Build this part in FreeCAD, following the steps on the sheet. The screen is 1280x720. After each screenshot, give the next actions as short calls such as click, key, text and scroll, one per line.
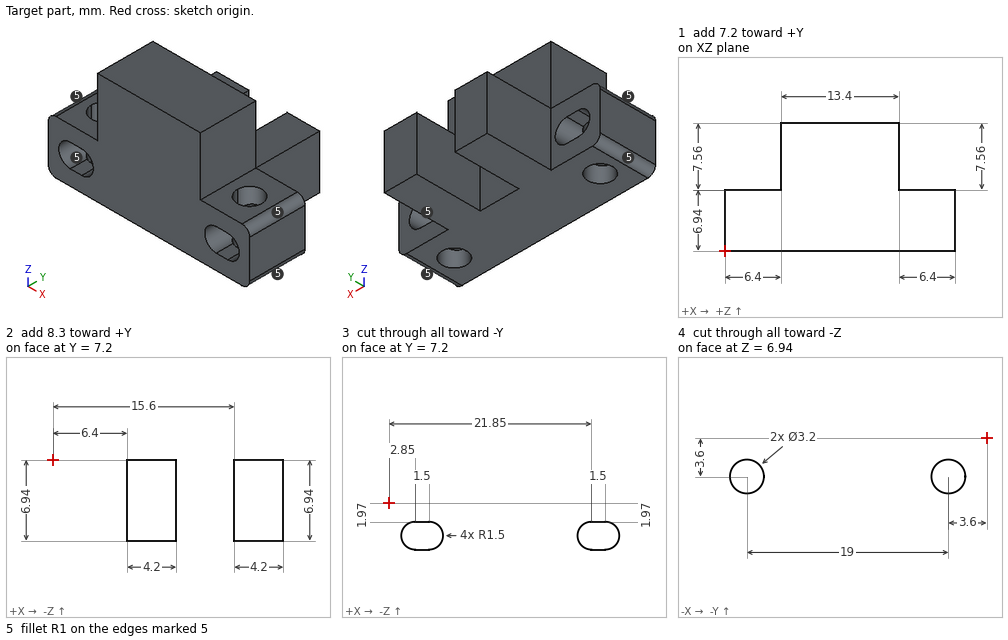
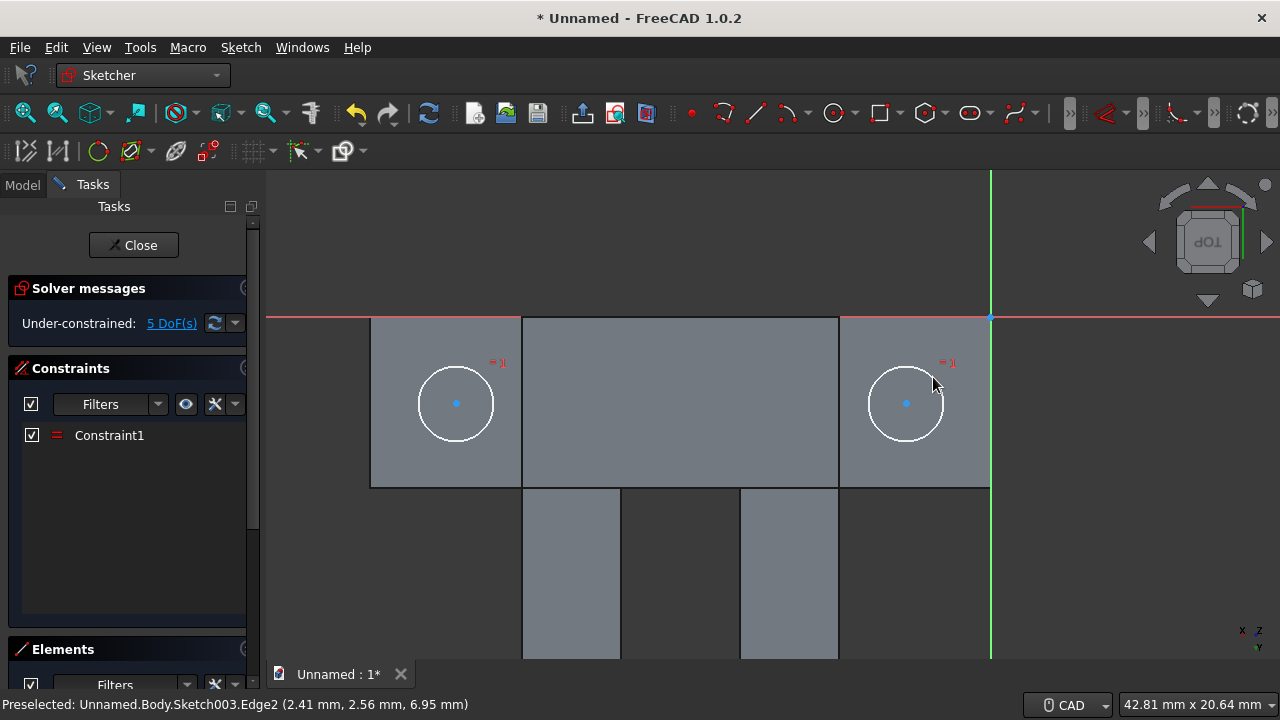
click(456, 404)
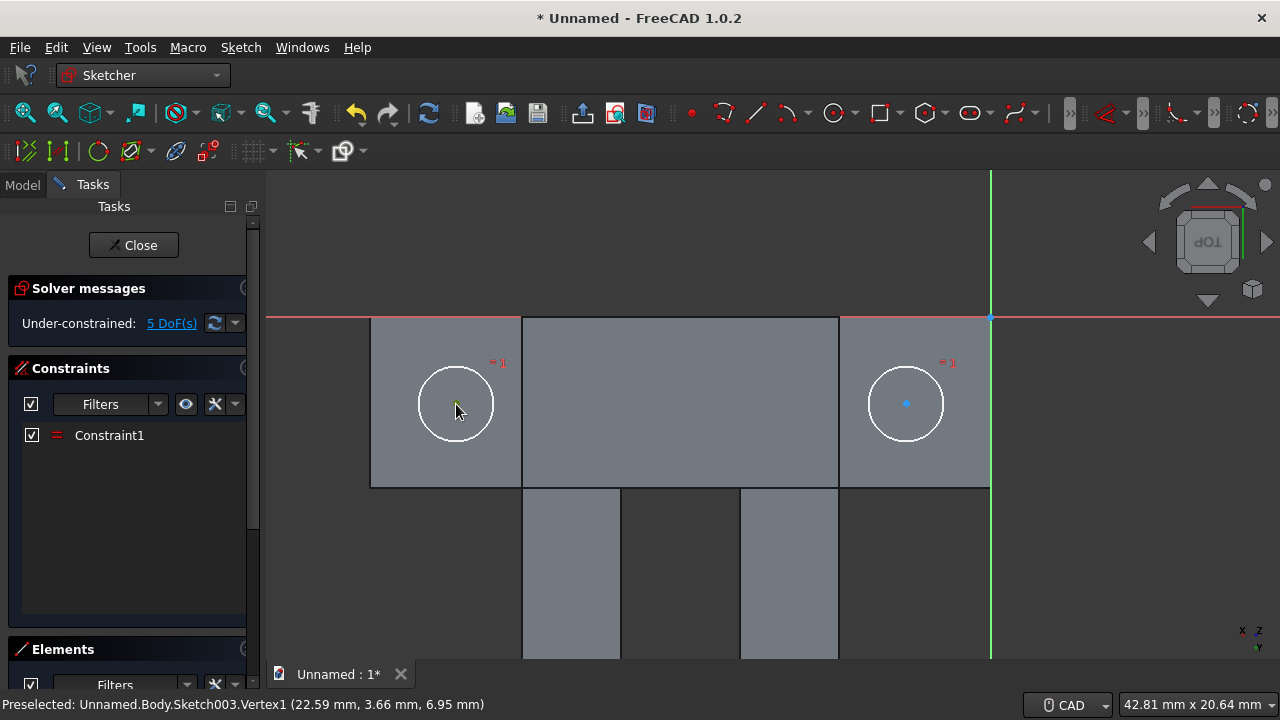
click(906, 404)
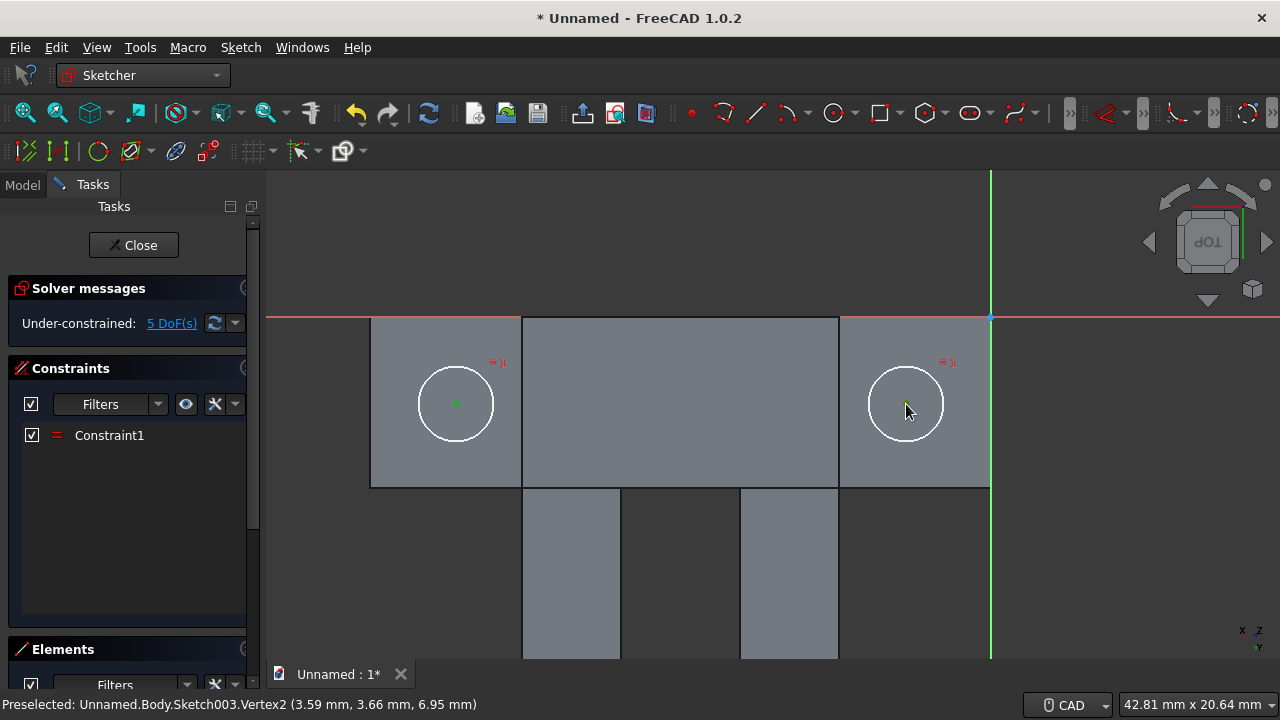
key(h)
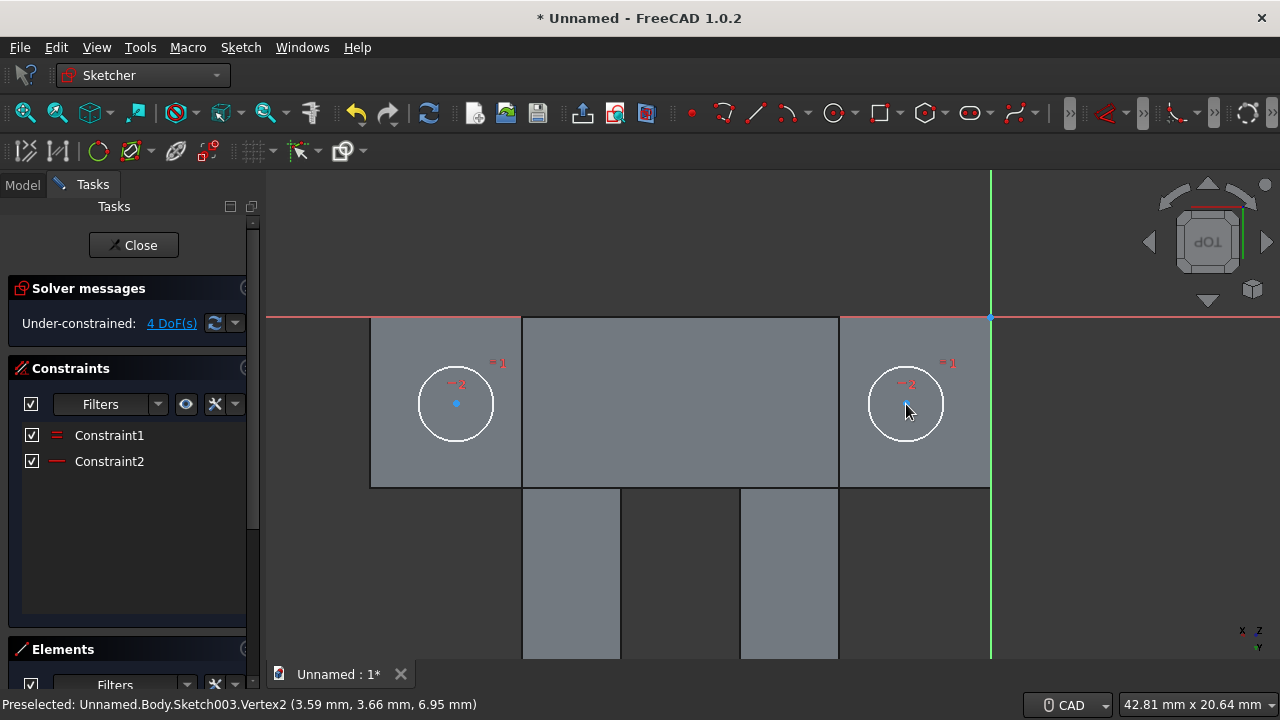
click(1106, 114)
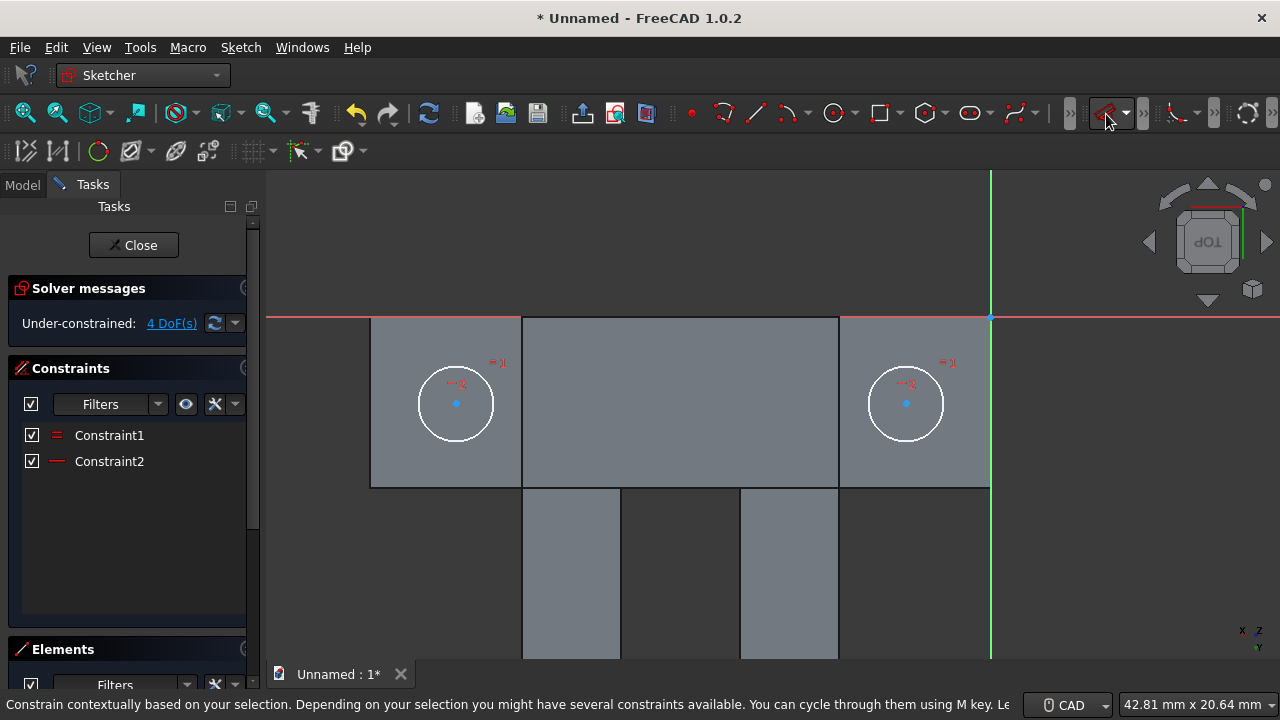
click(482, 377)
click(504, 354)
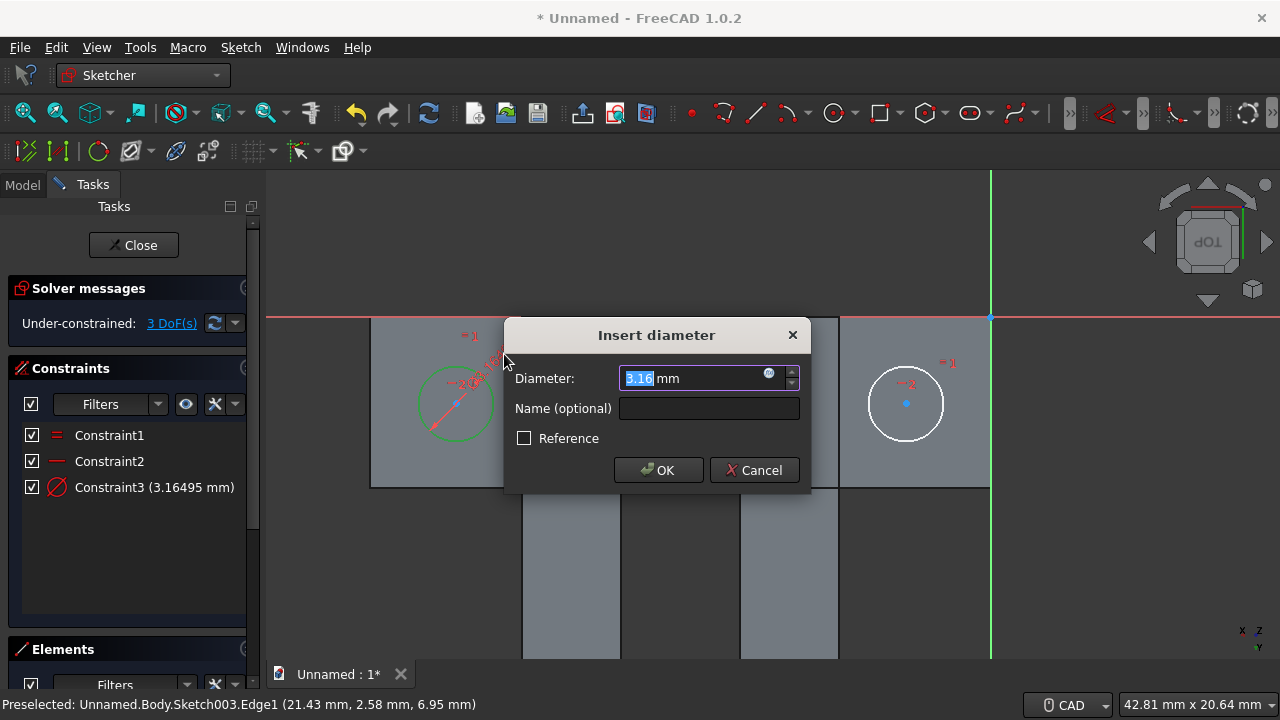
text(3.2)
key(Return)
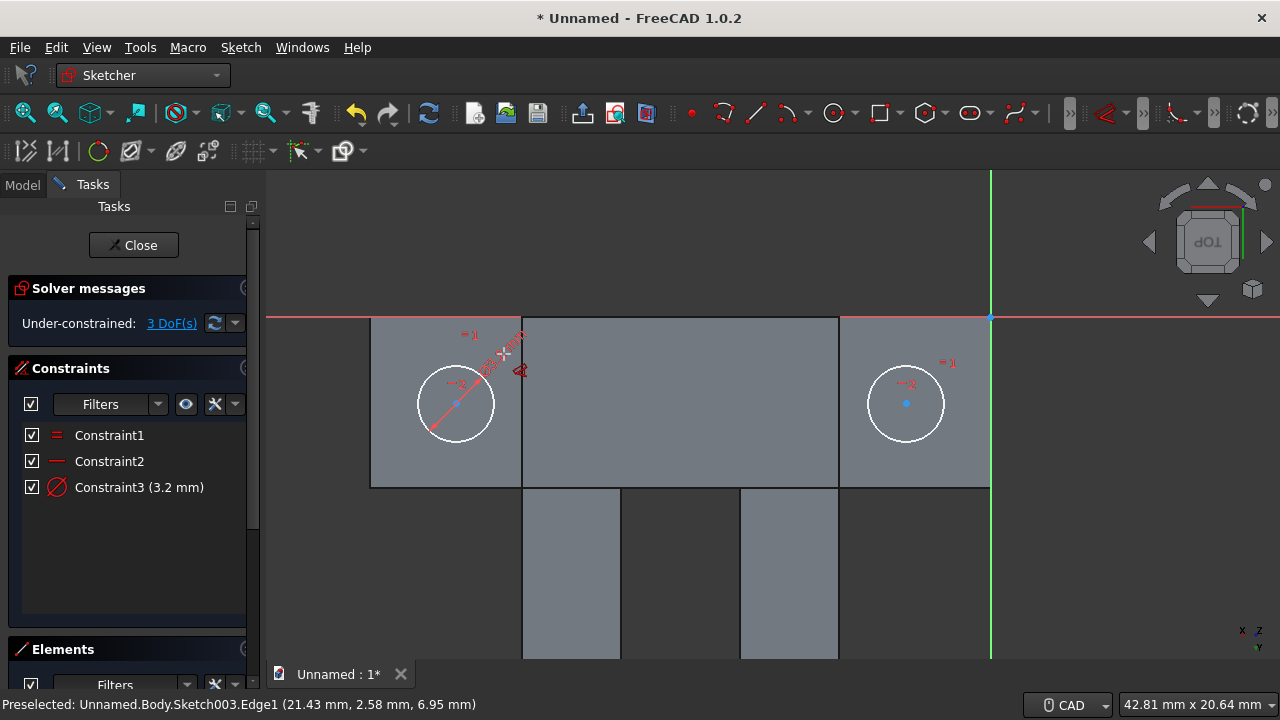
click(456, 404)
click(1025, 361)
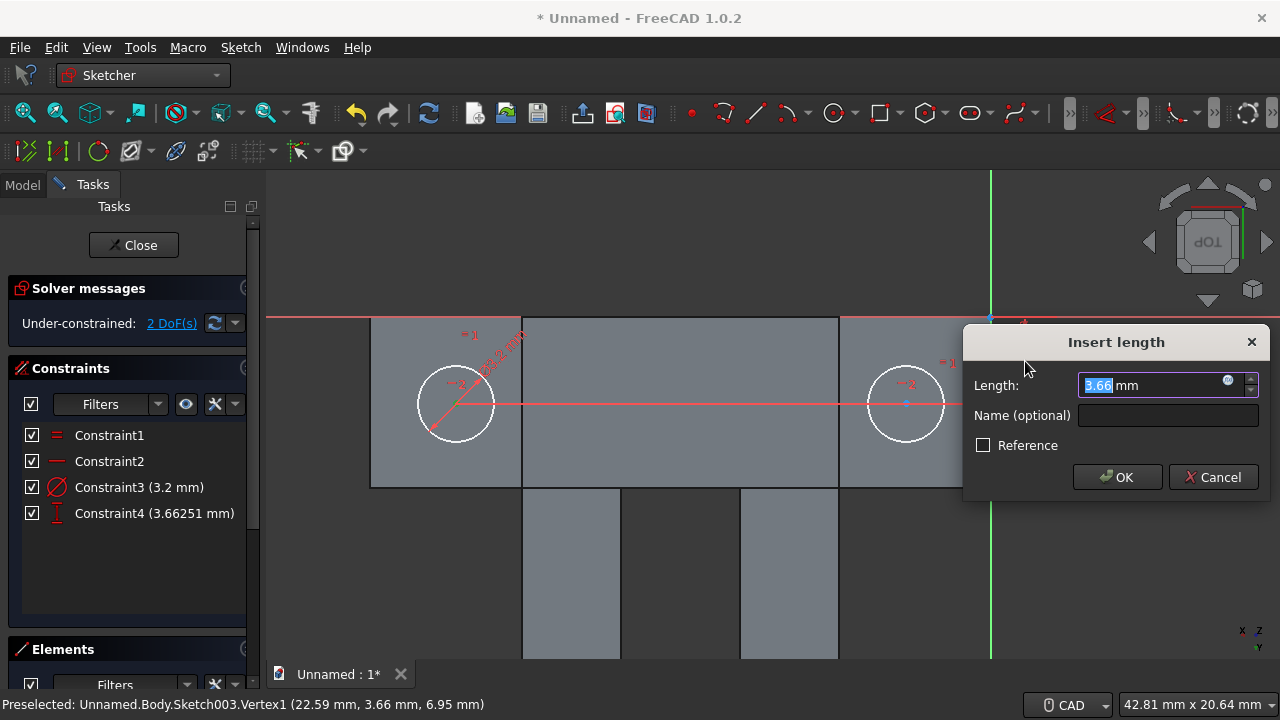
text(3.6)
key(Return)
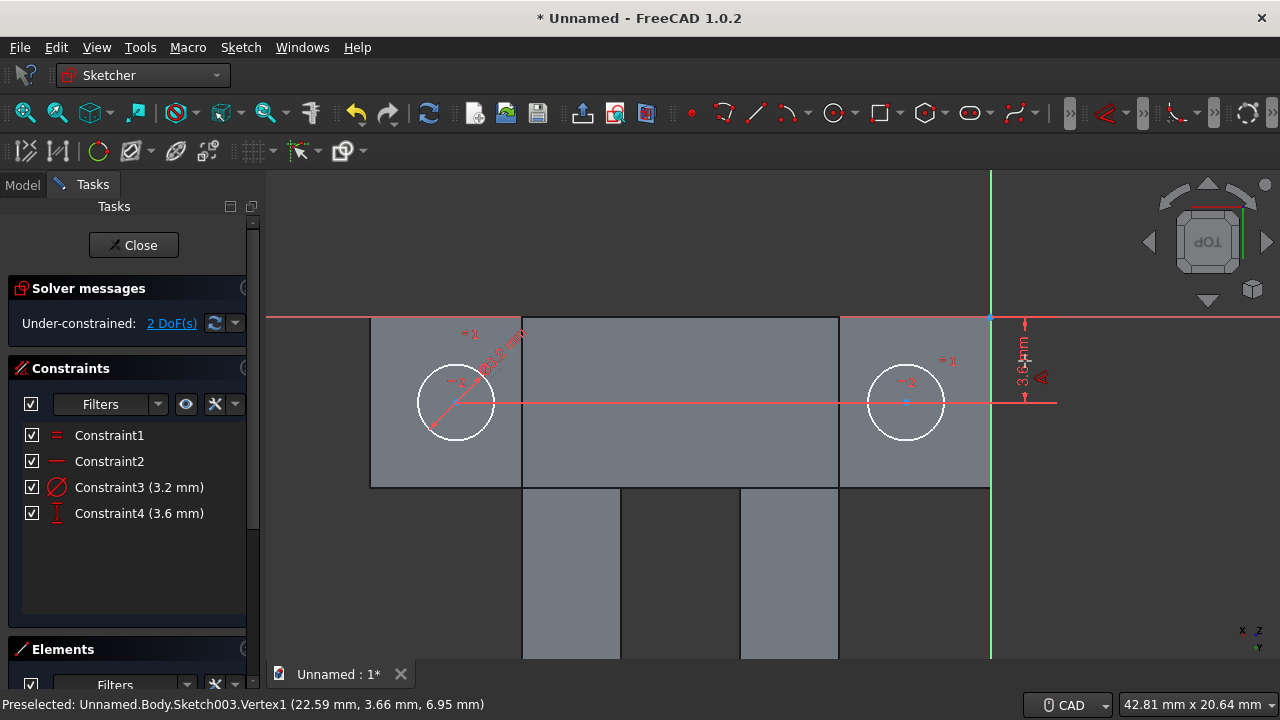
click(906, 403)
click(948, 283)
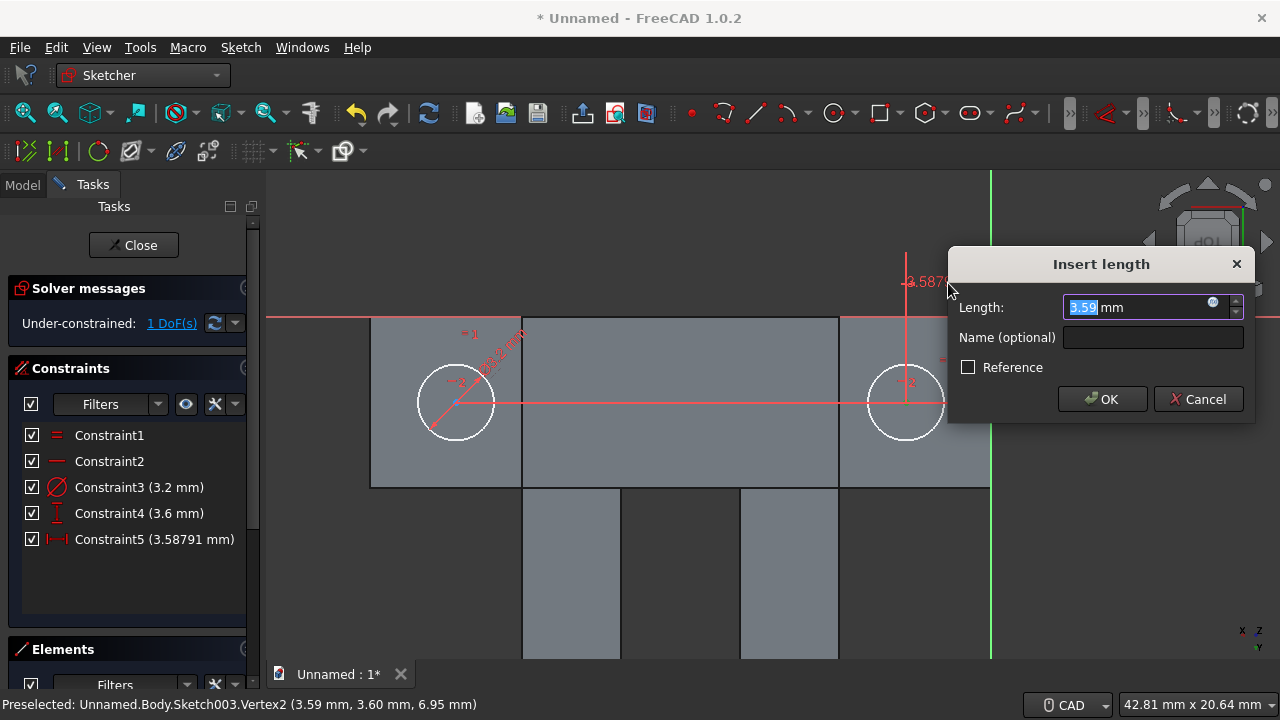
text(3.6)
key(Return)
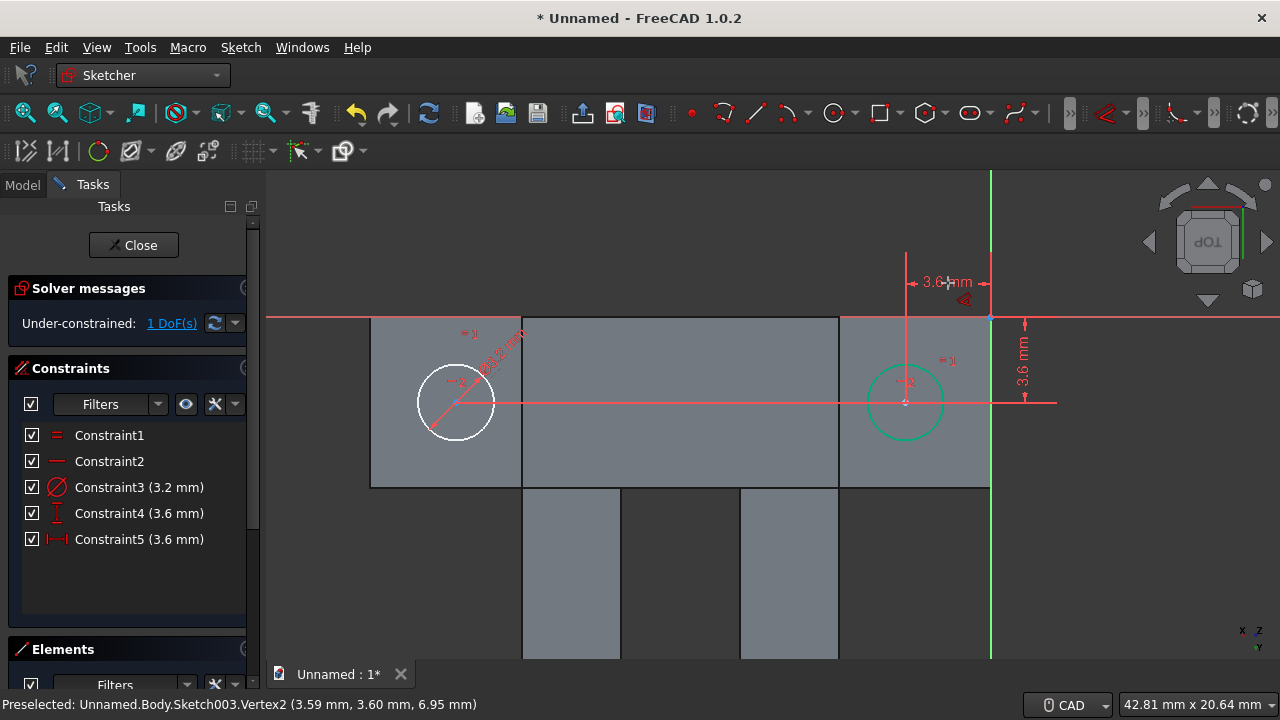
click(456, 403)